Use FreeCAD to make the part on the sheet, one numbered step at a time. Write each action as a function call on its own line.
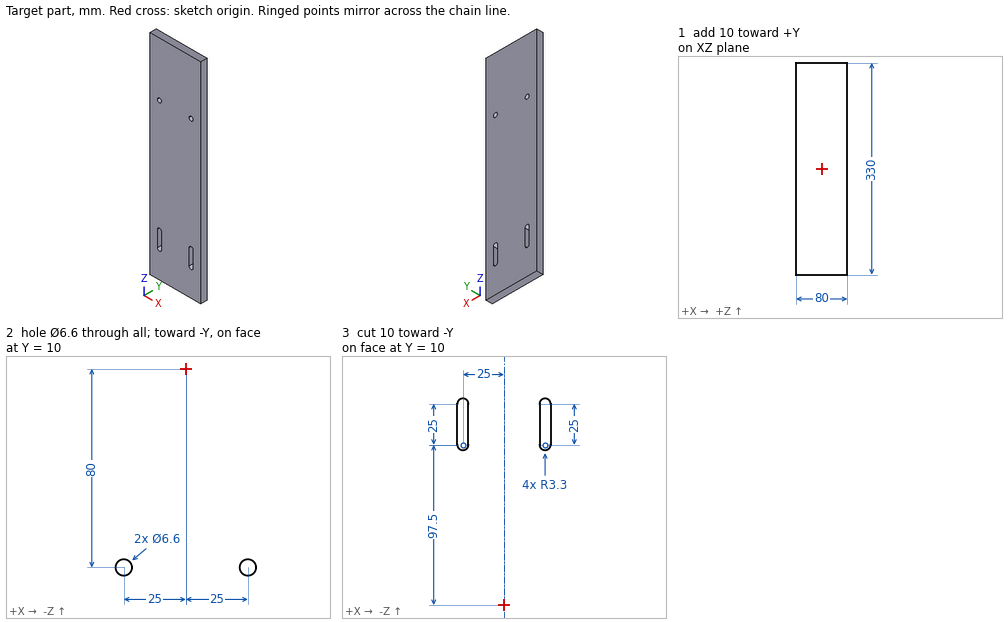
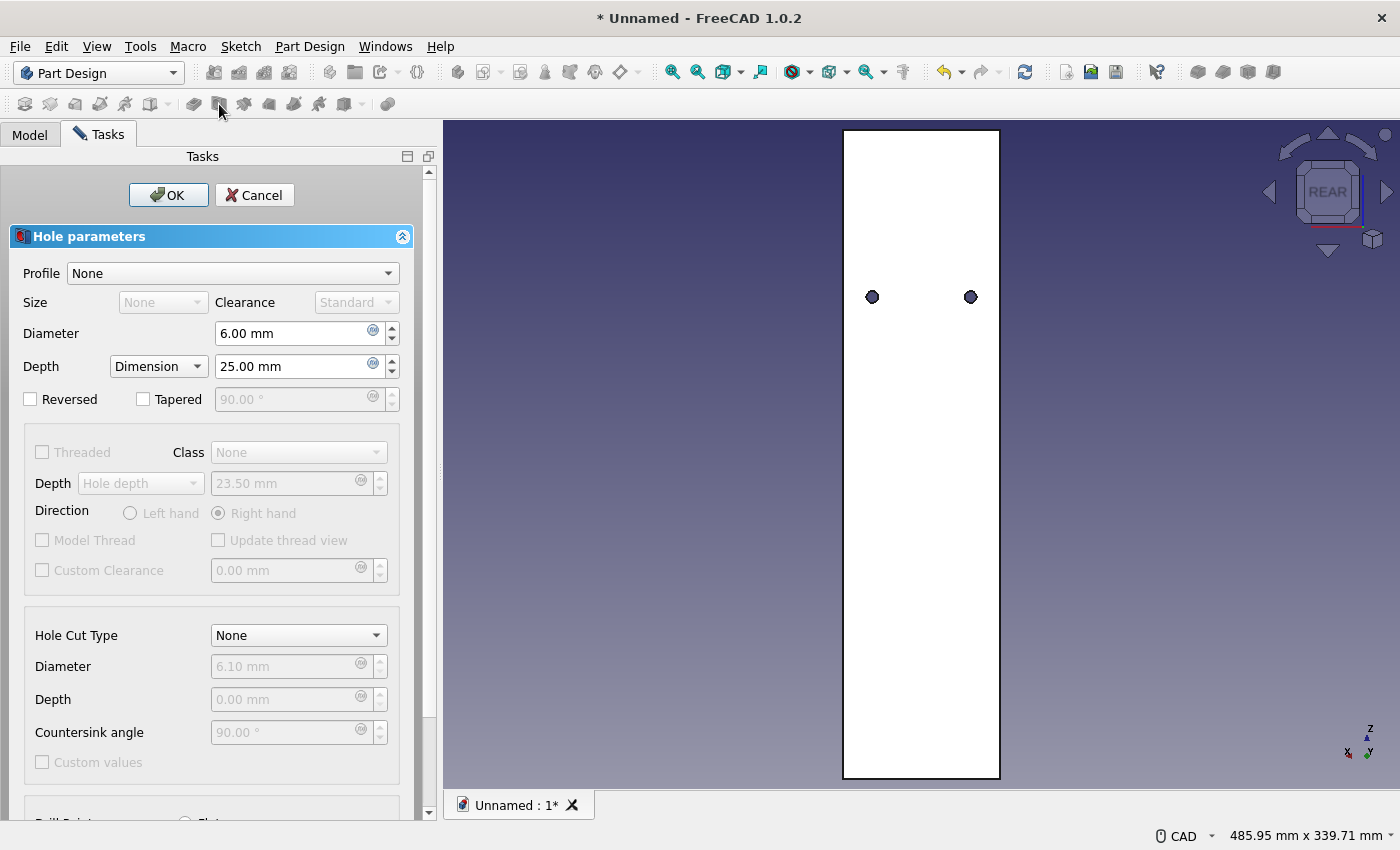
triple_click(300, 334)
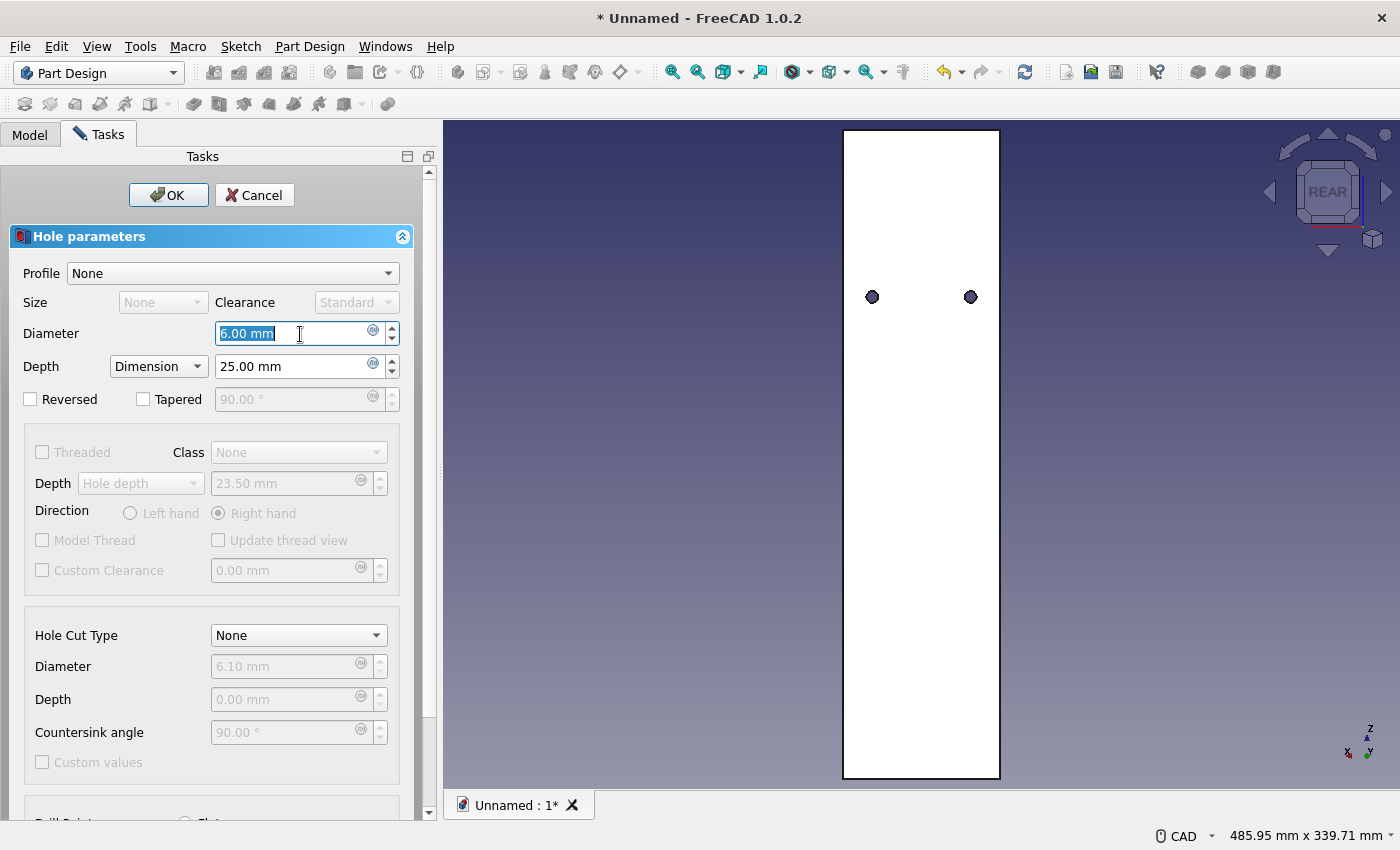
text(6.6)
key(Tab)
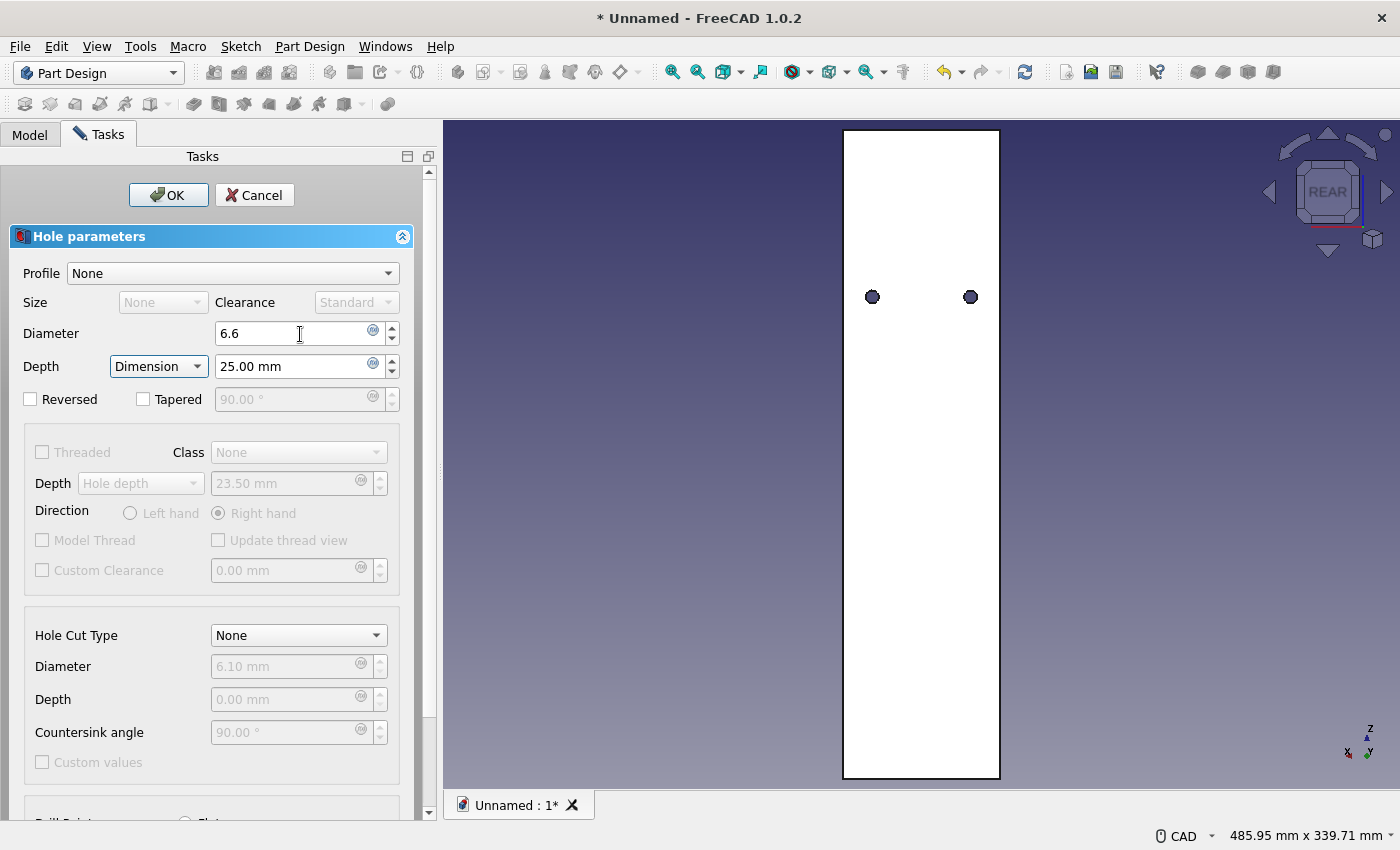
click(160, 366)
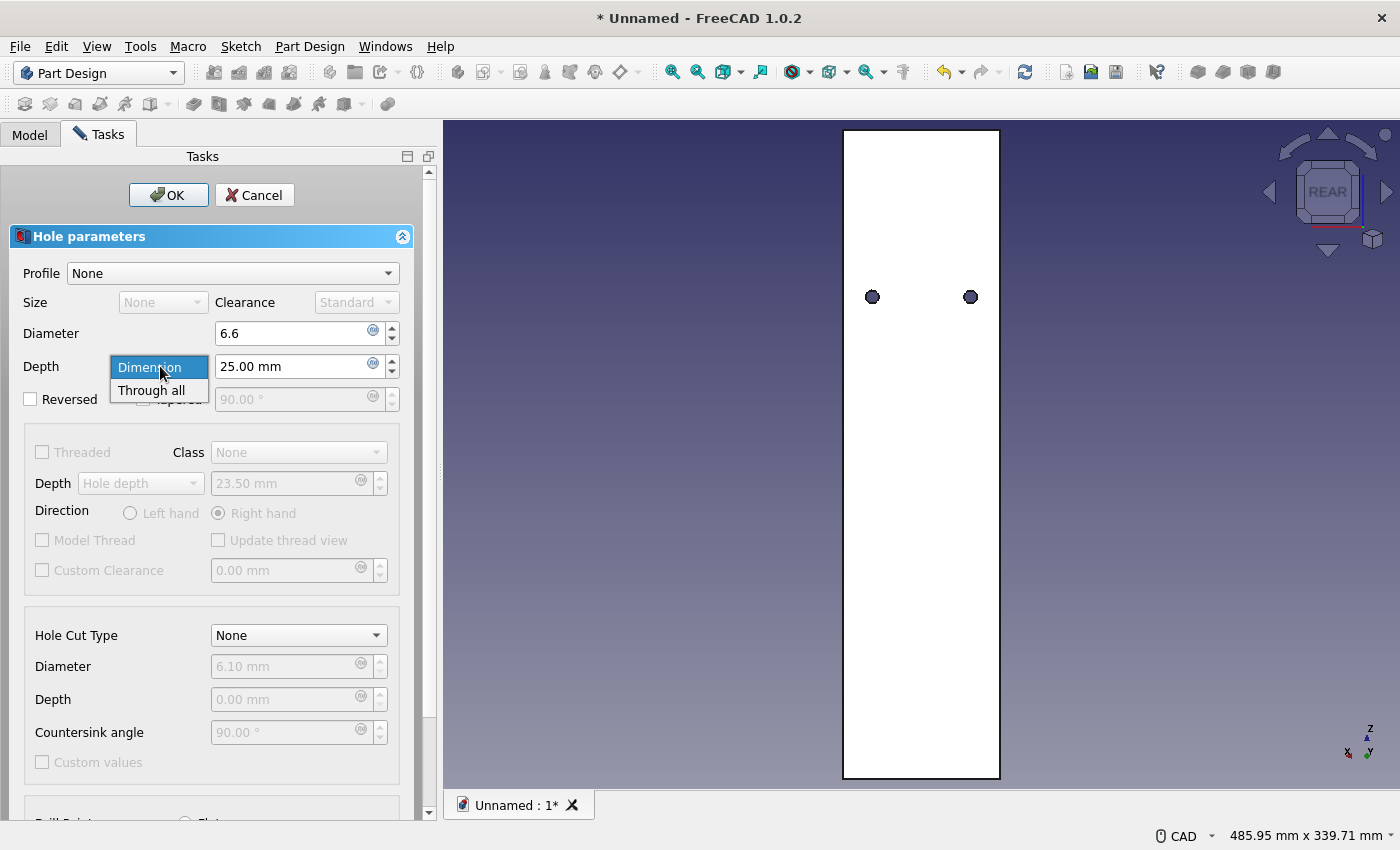
click(158, 390)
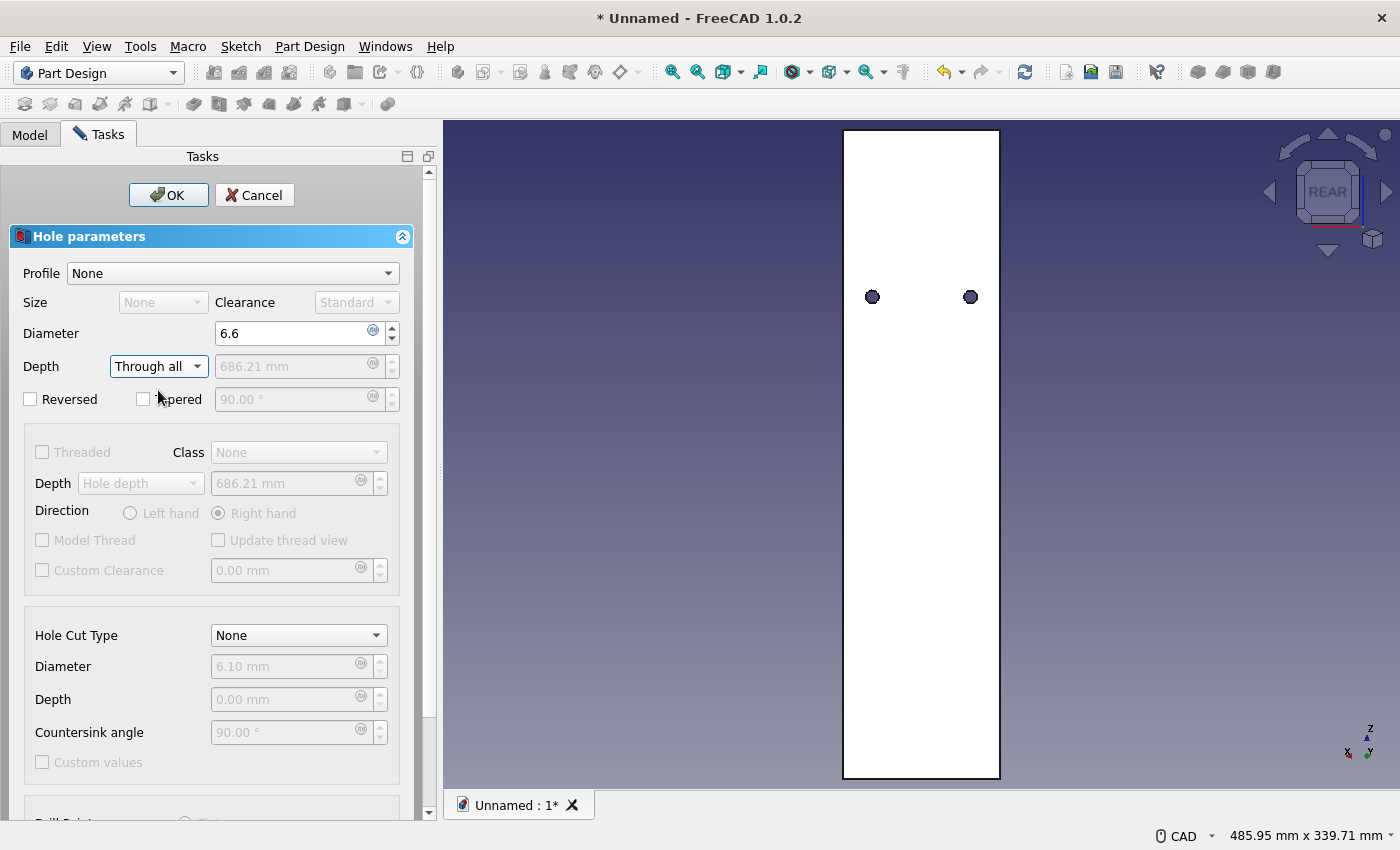
click(169, 195)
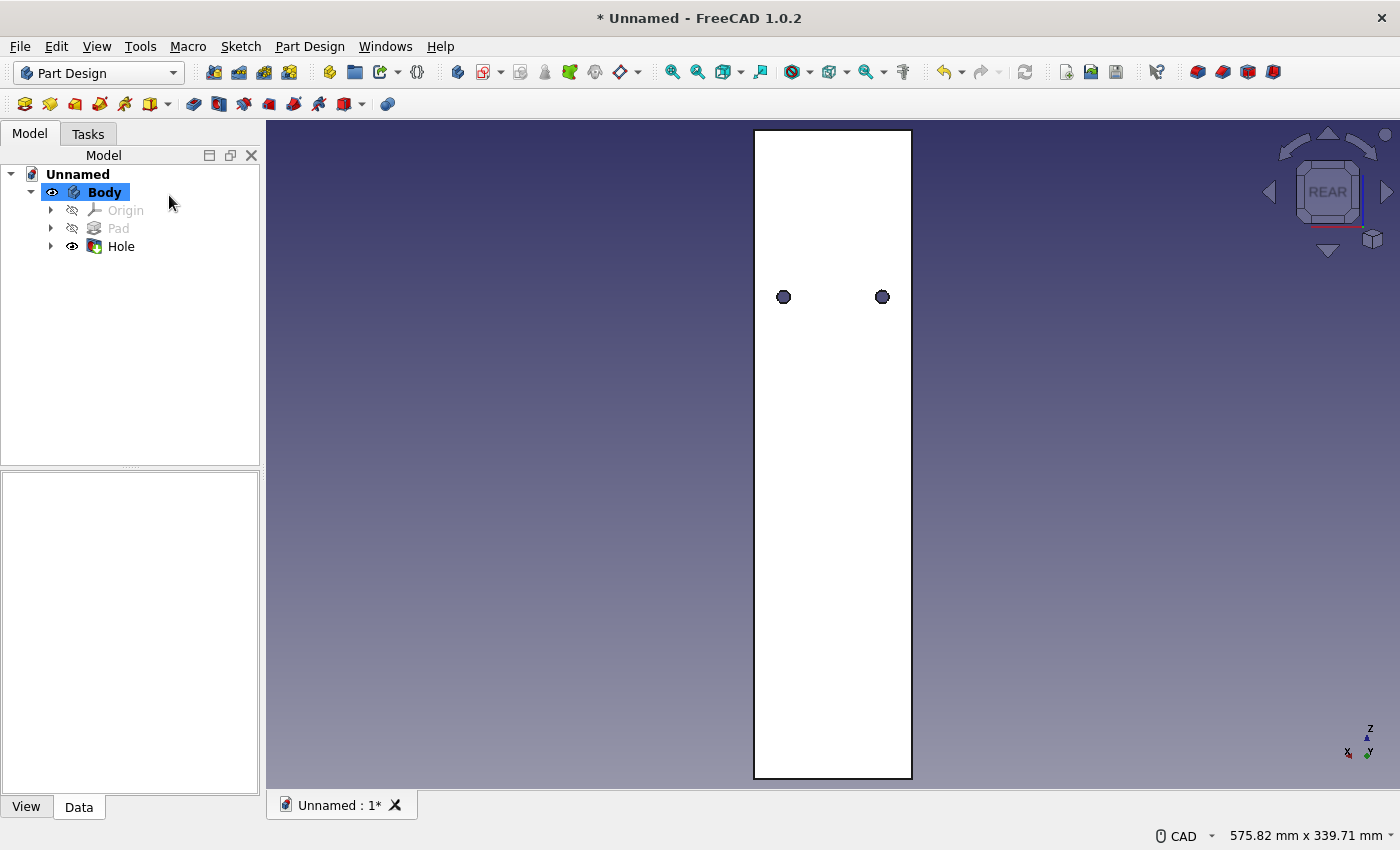
click(833, 454)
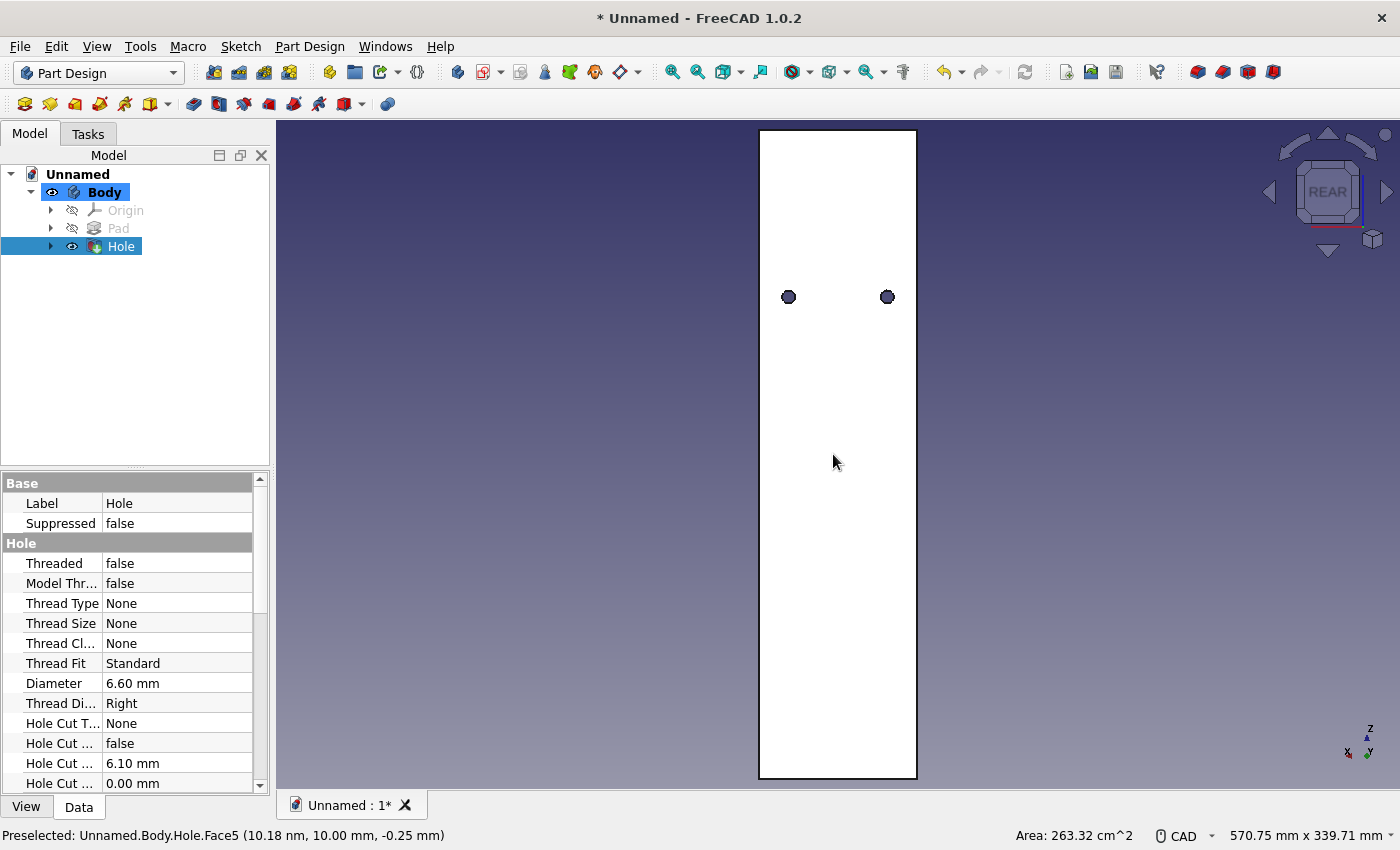
click(482, 72)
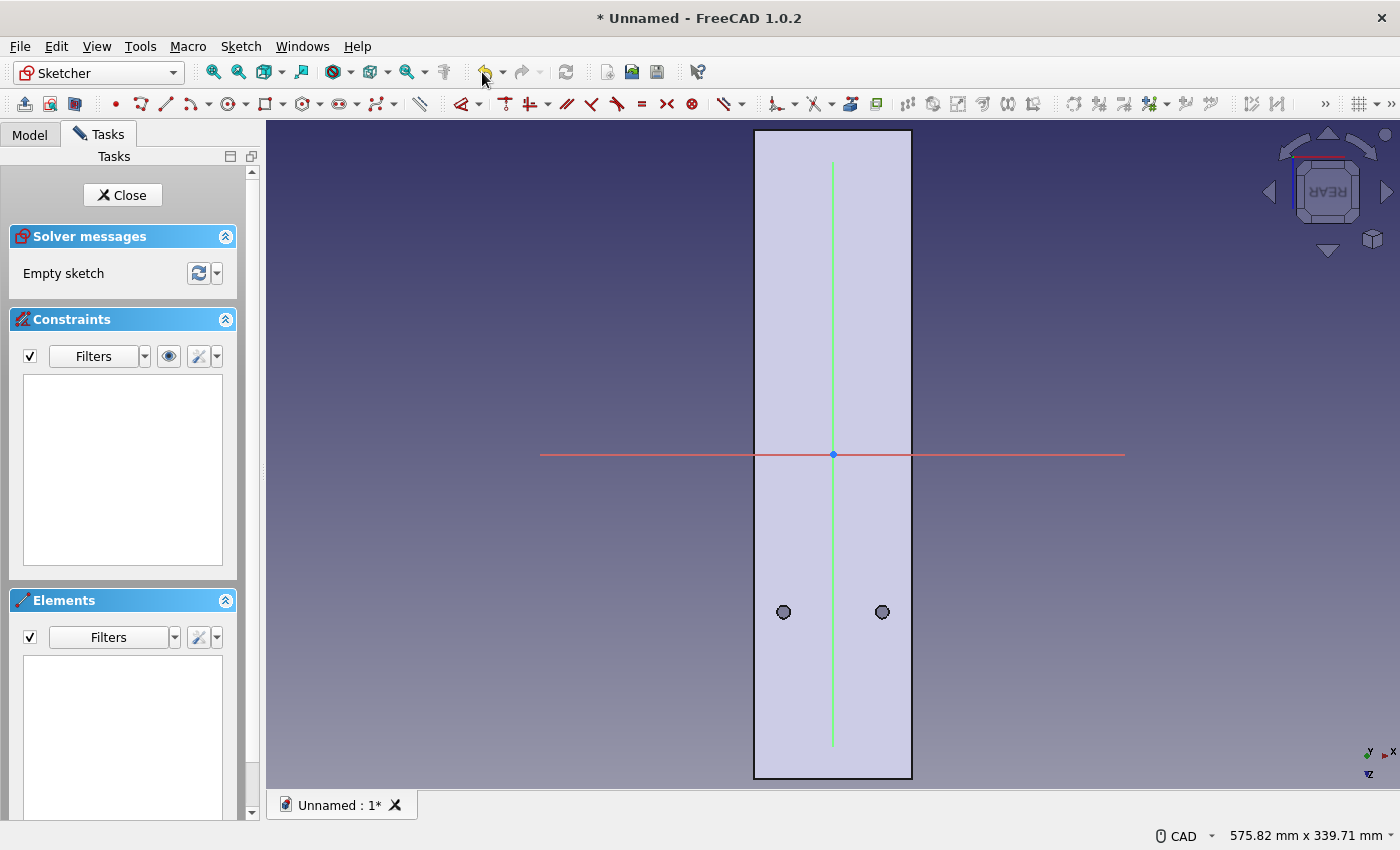
scroll(916, 180, up, 3)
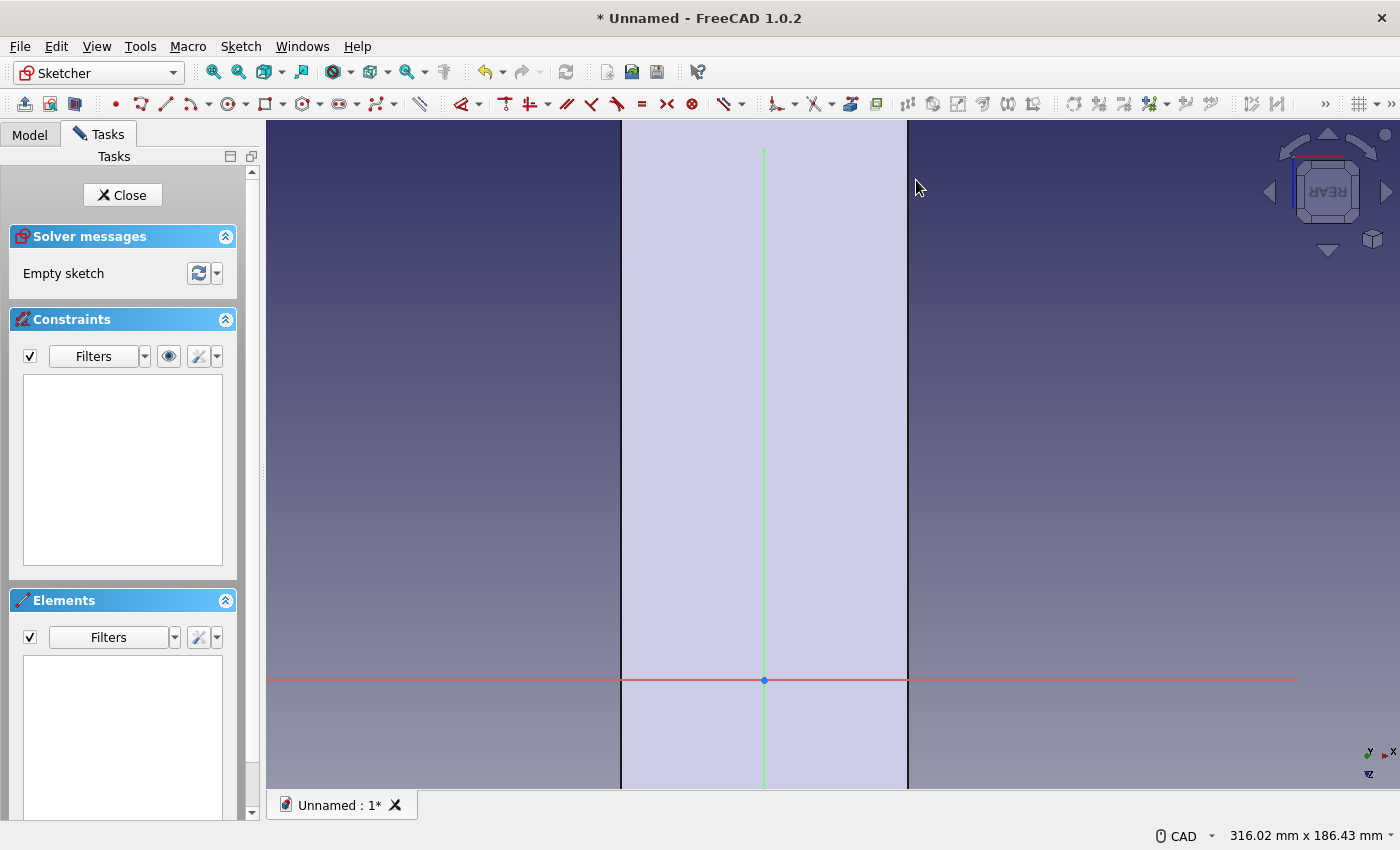
key(g)
key(s)